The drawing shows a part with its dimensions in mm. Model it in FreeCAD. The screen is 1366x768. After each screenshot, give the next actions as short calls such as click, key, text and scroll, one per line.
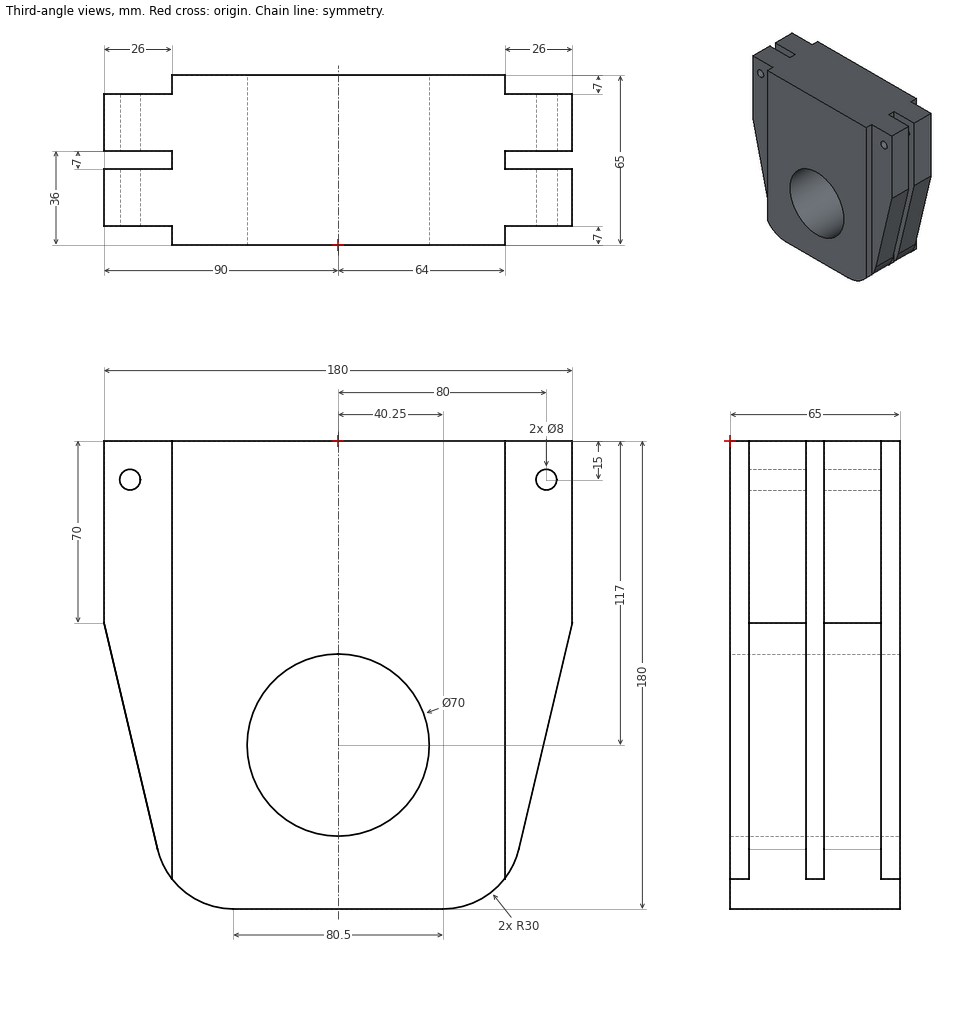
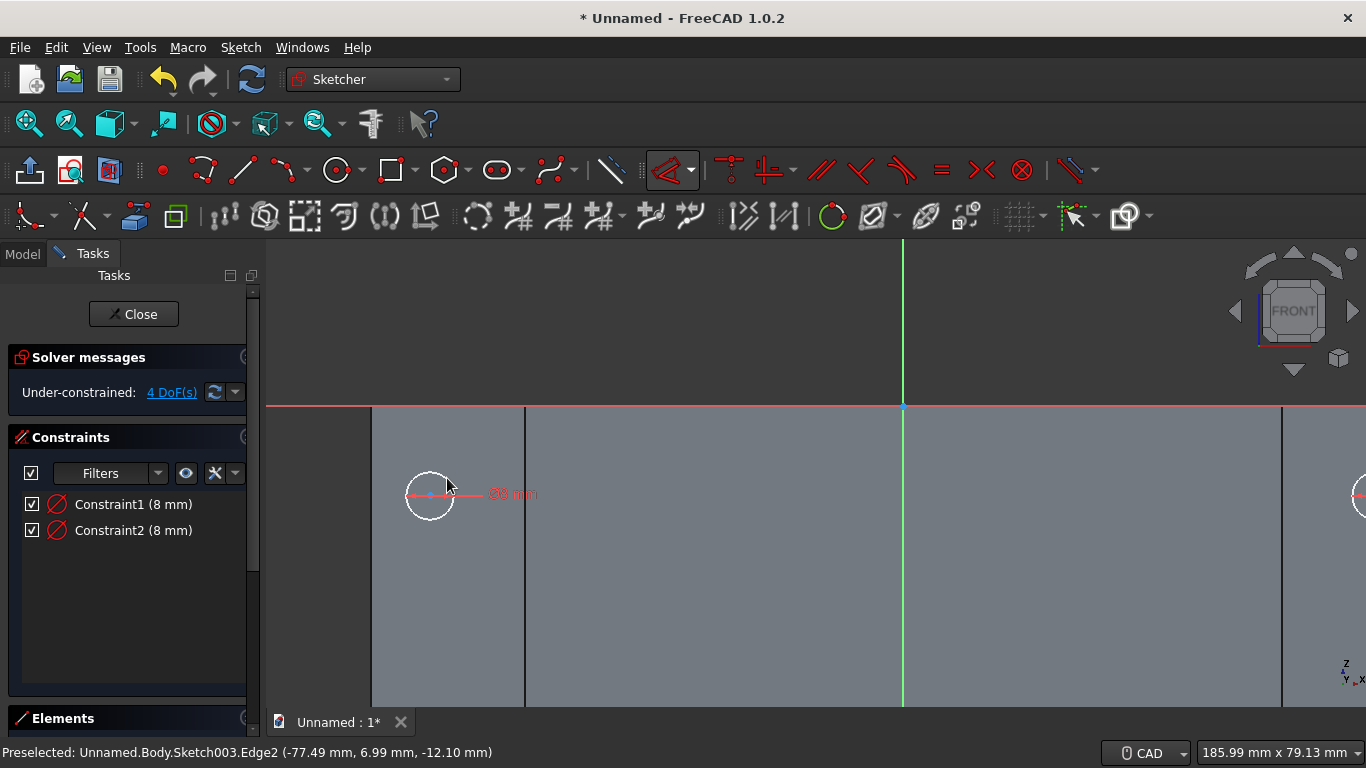
scroll(431, 495, down, 2)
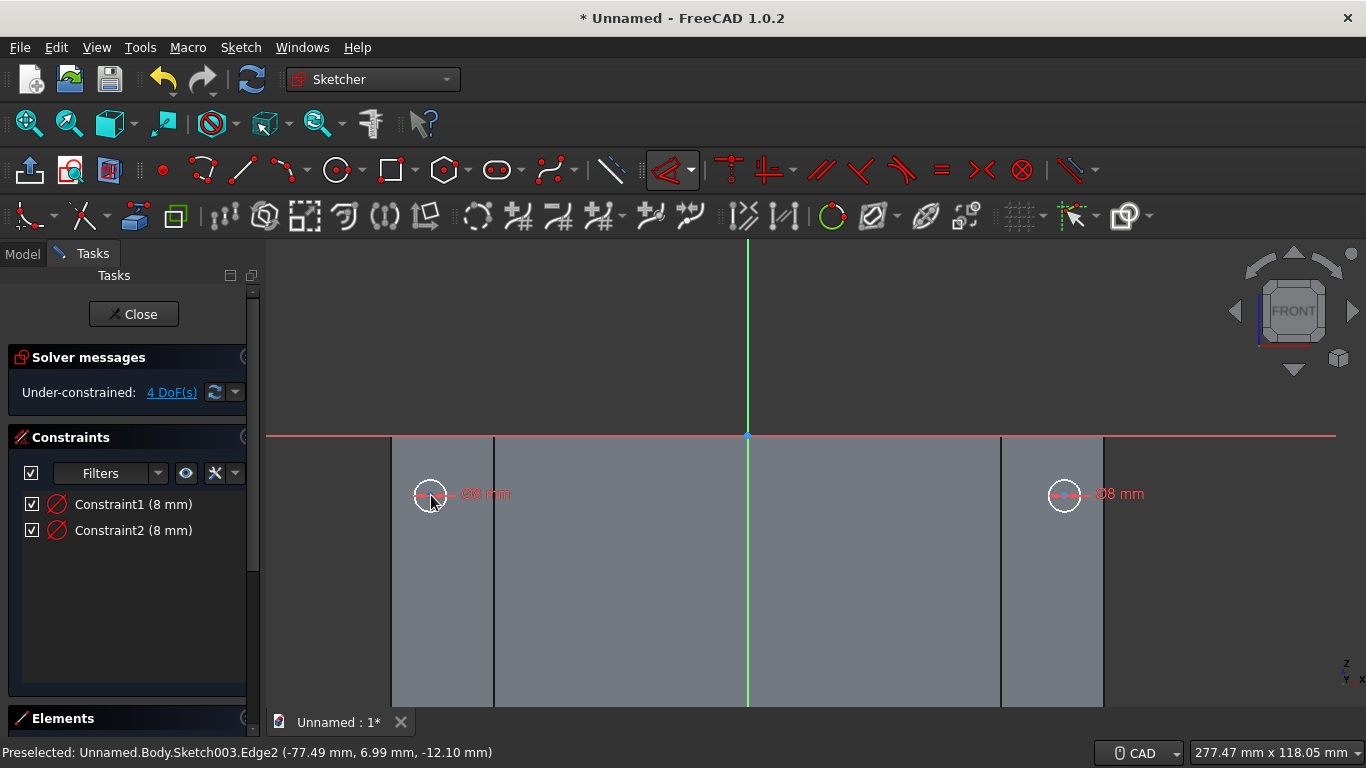
click(1065, 496)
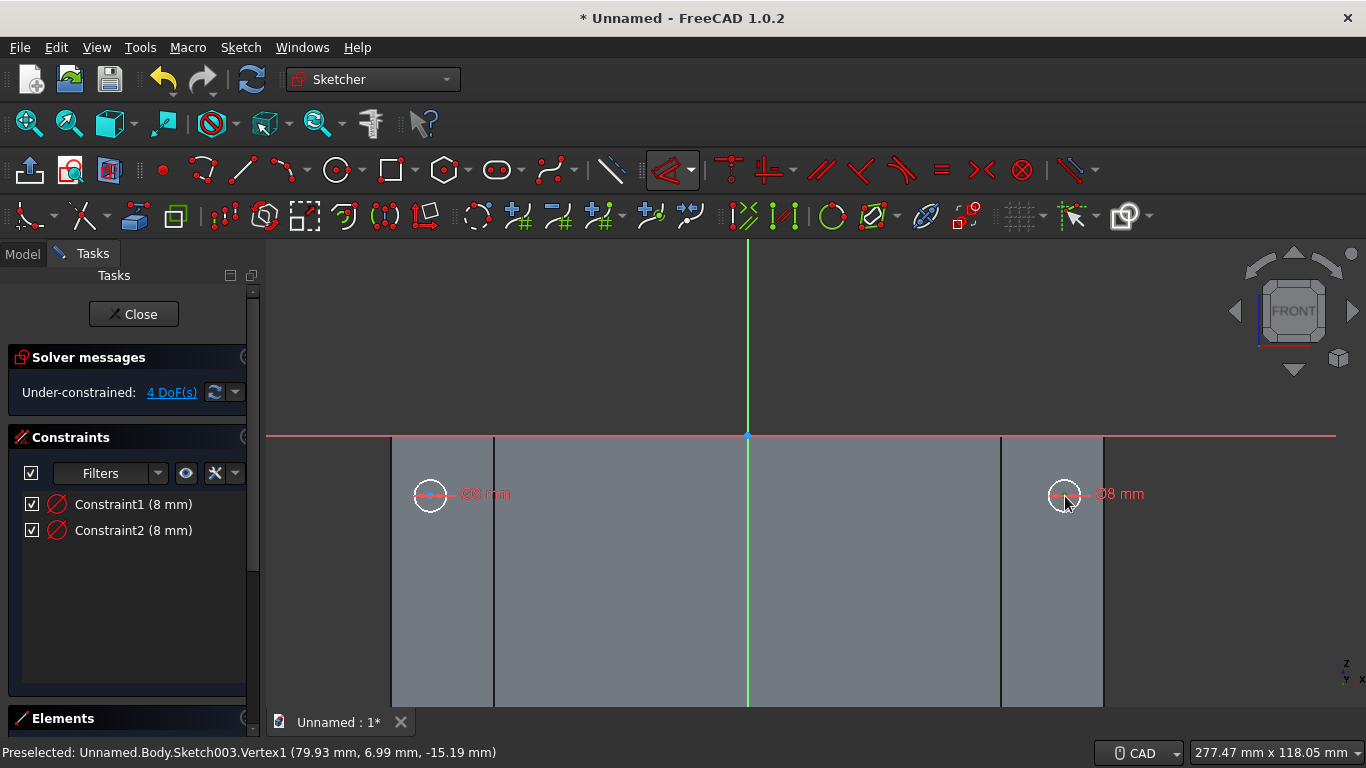
click(430, 496)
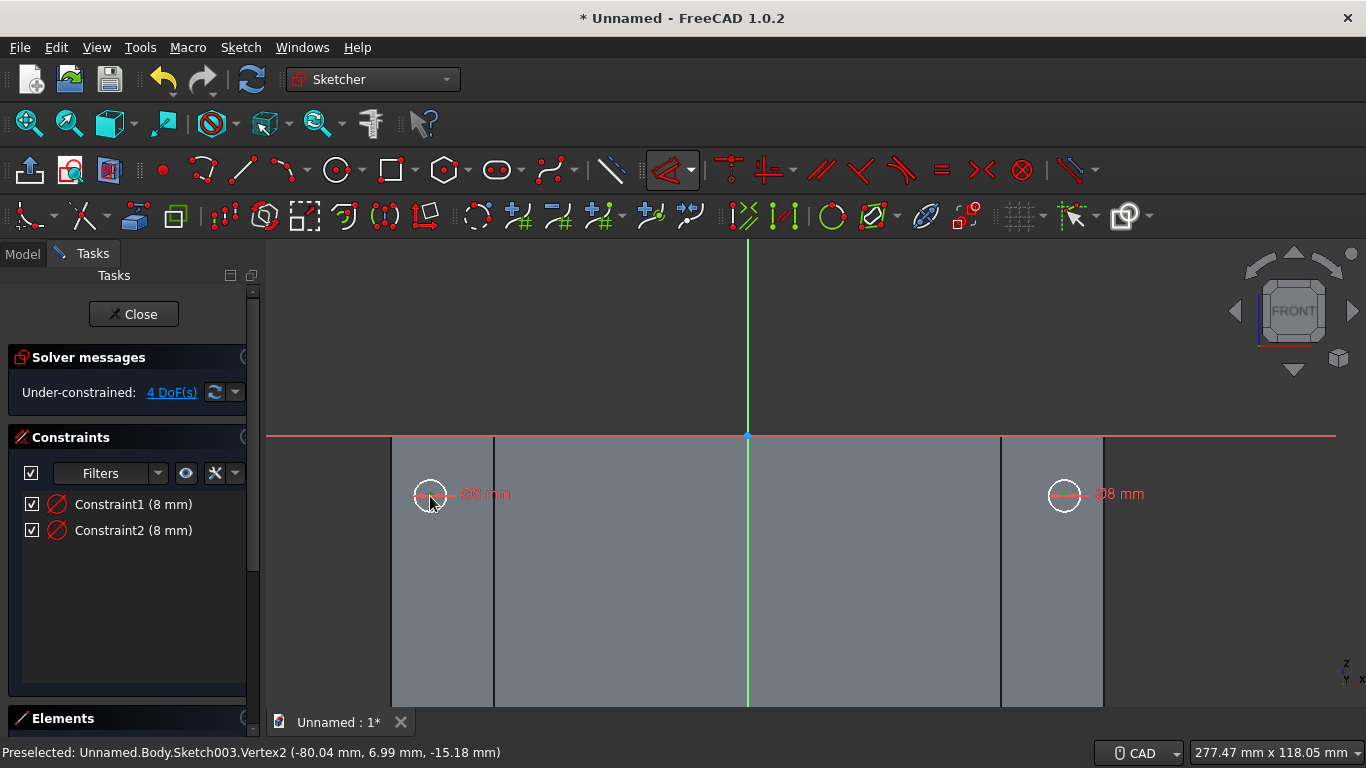
click(748, 650)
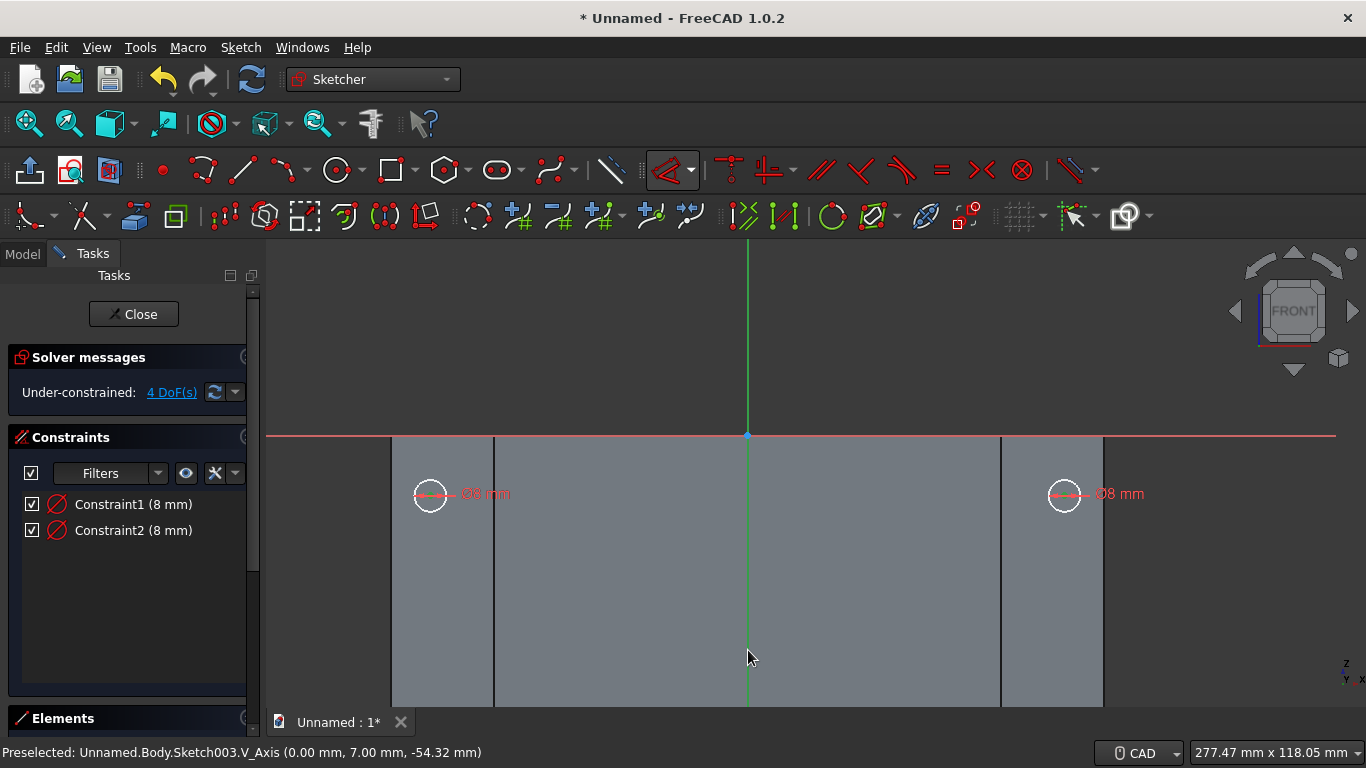
click(982, 170)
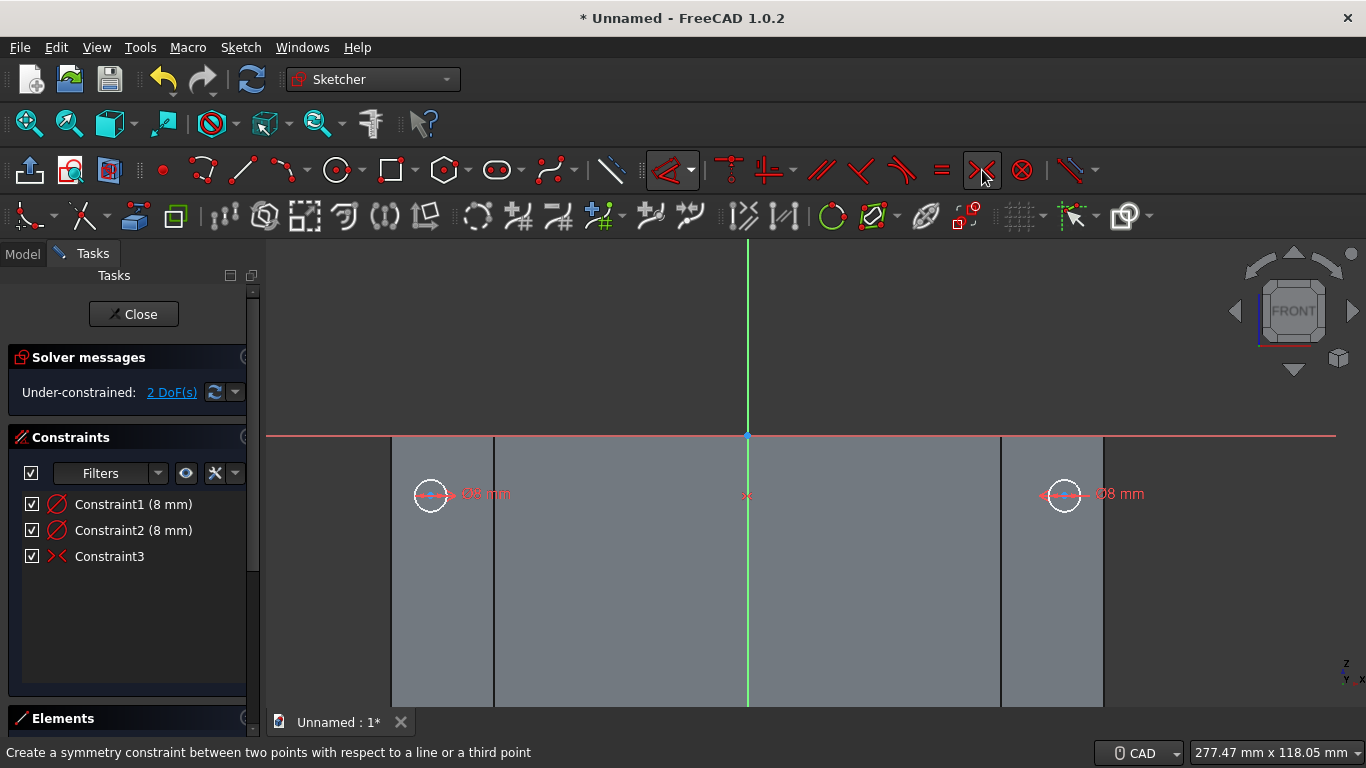
click(1065, 496)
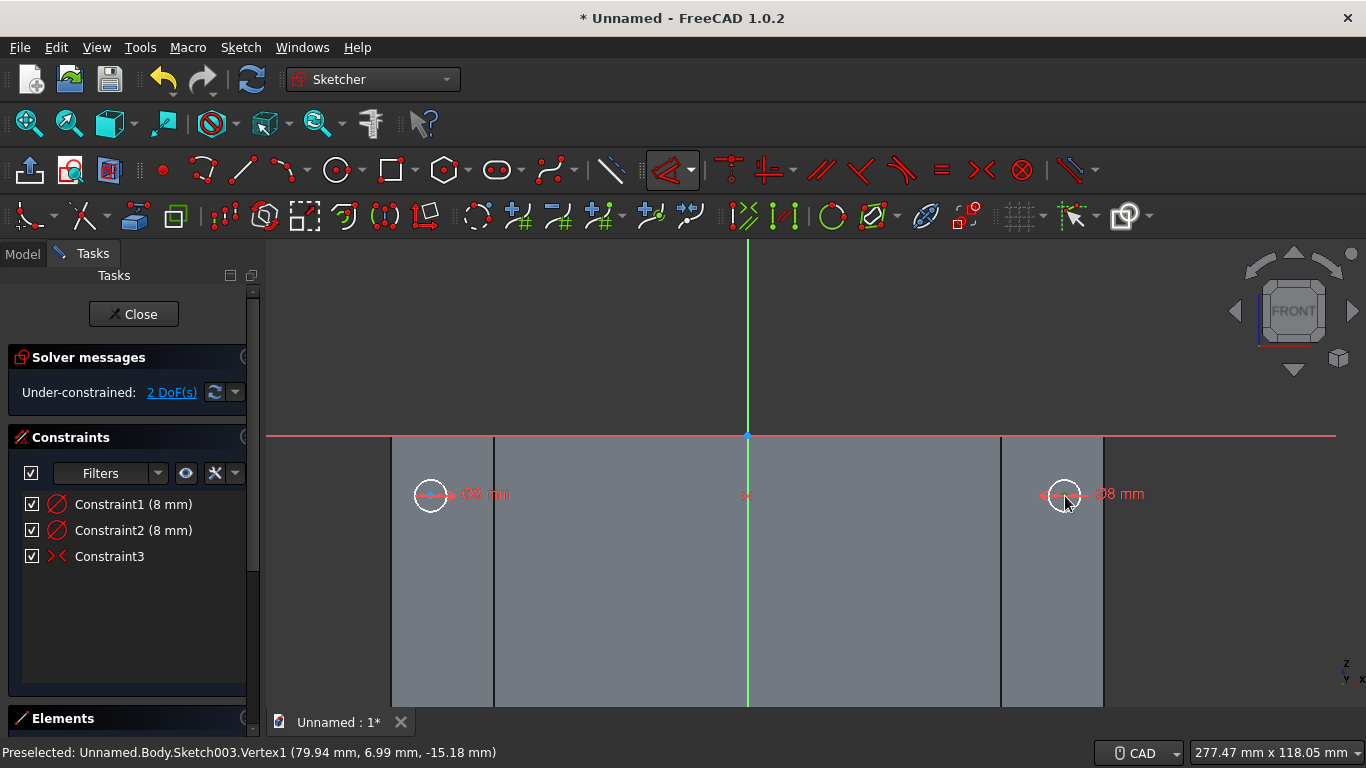
key(l)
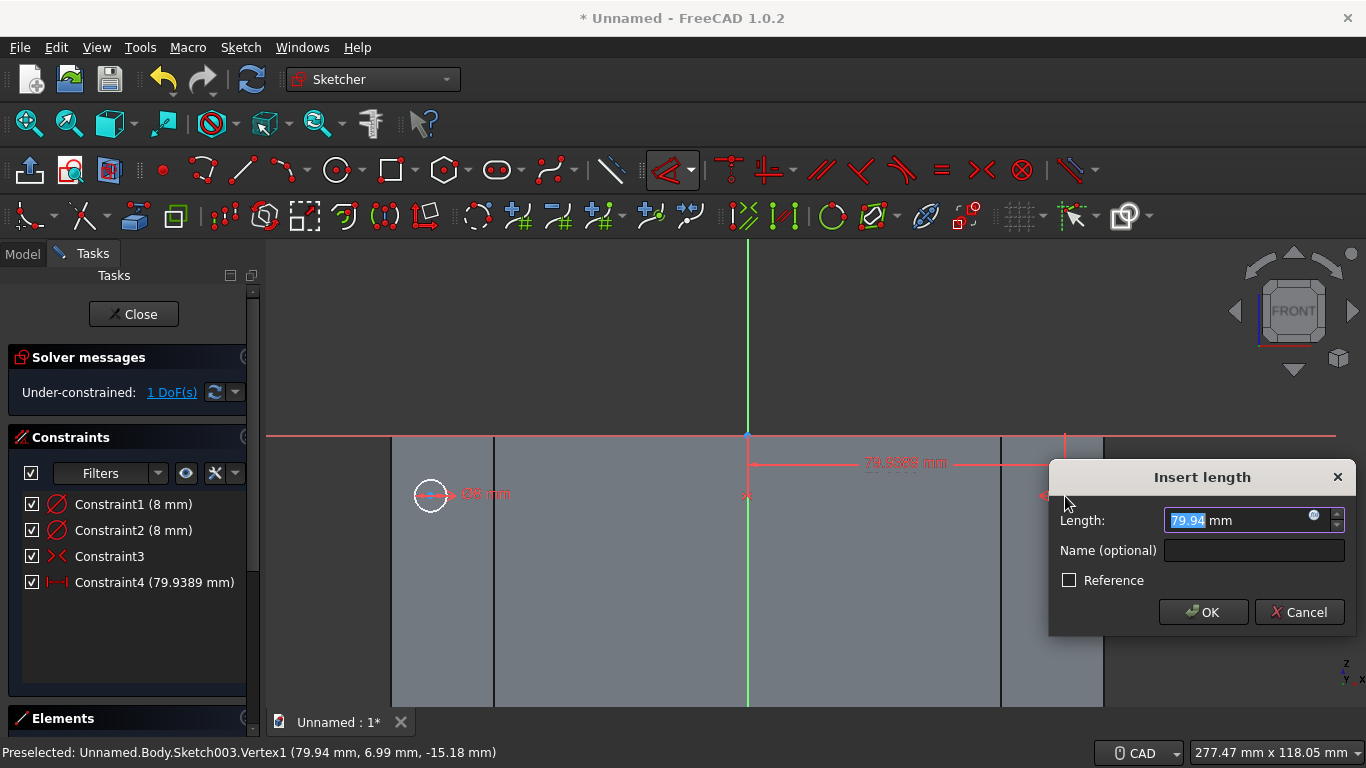
text(80)
key(Return)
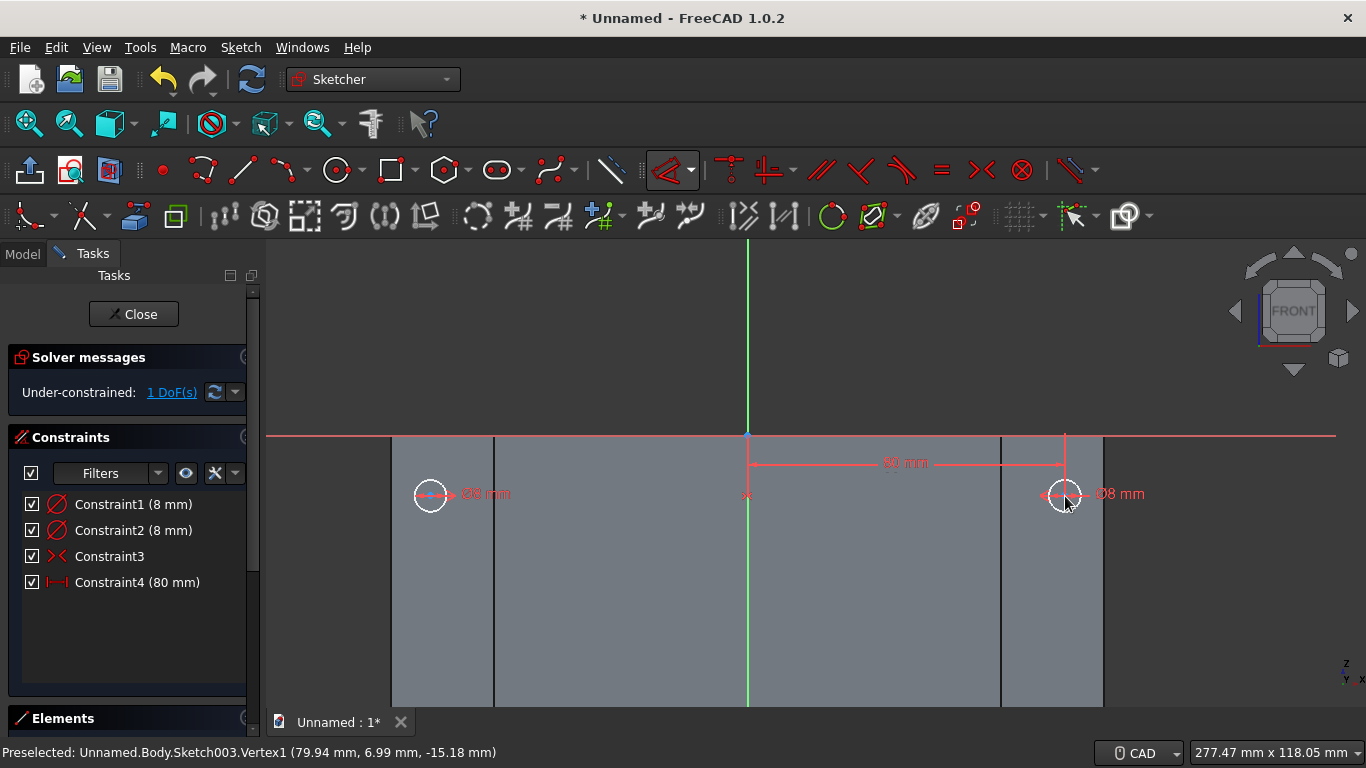
click(1065, 496)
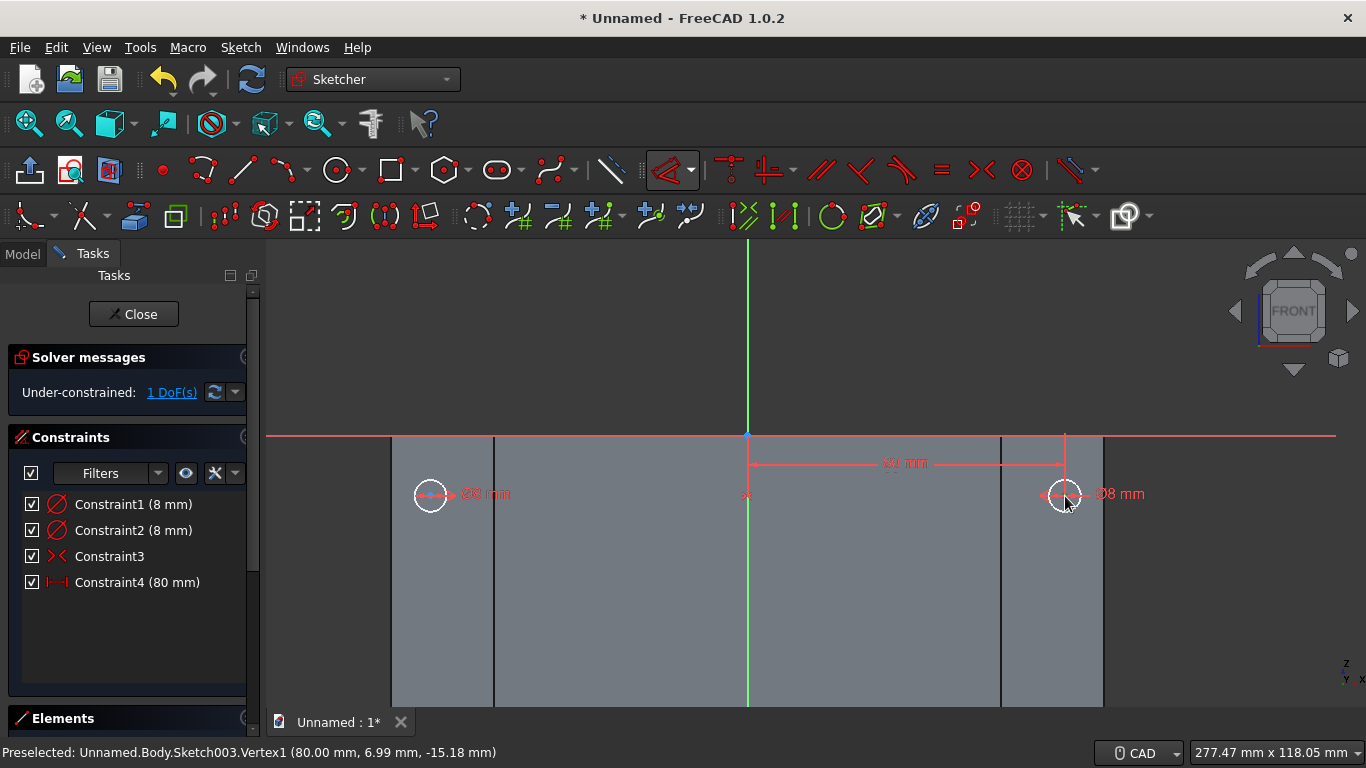
click(694, 170)